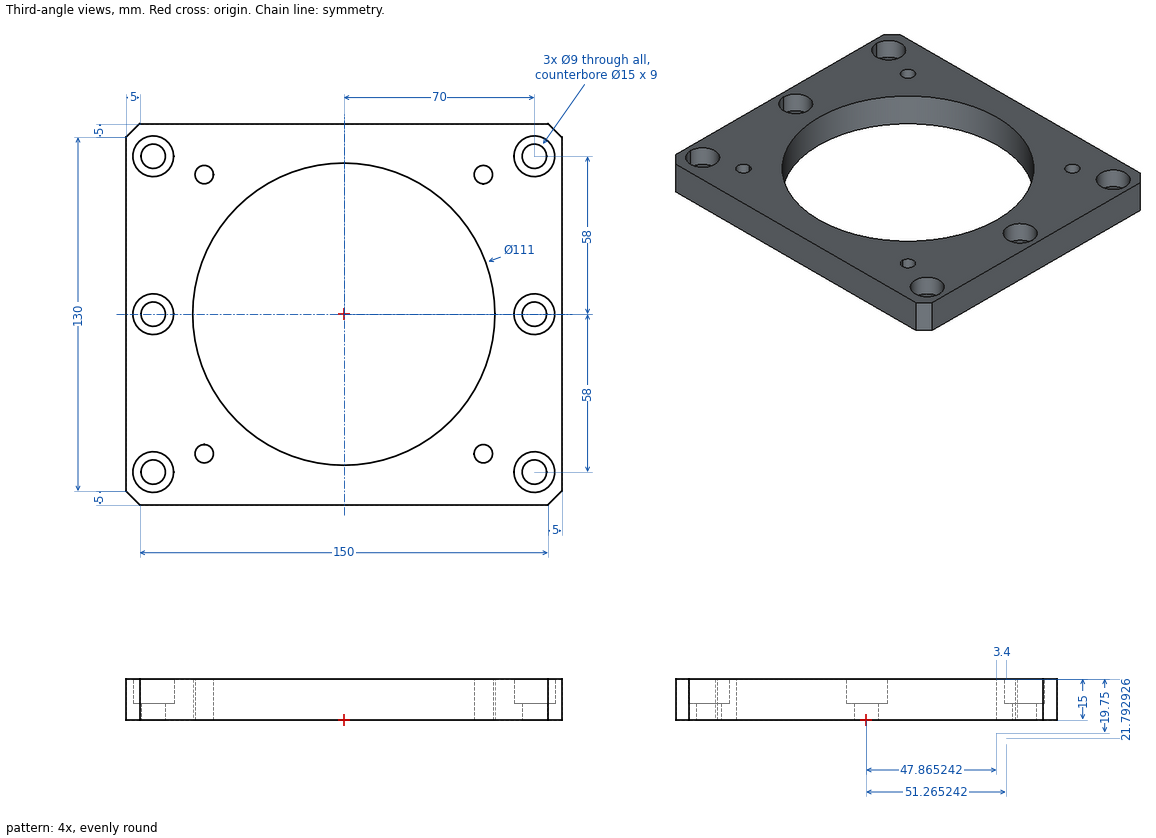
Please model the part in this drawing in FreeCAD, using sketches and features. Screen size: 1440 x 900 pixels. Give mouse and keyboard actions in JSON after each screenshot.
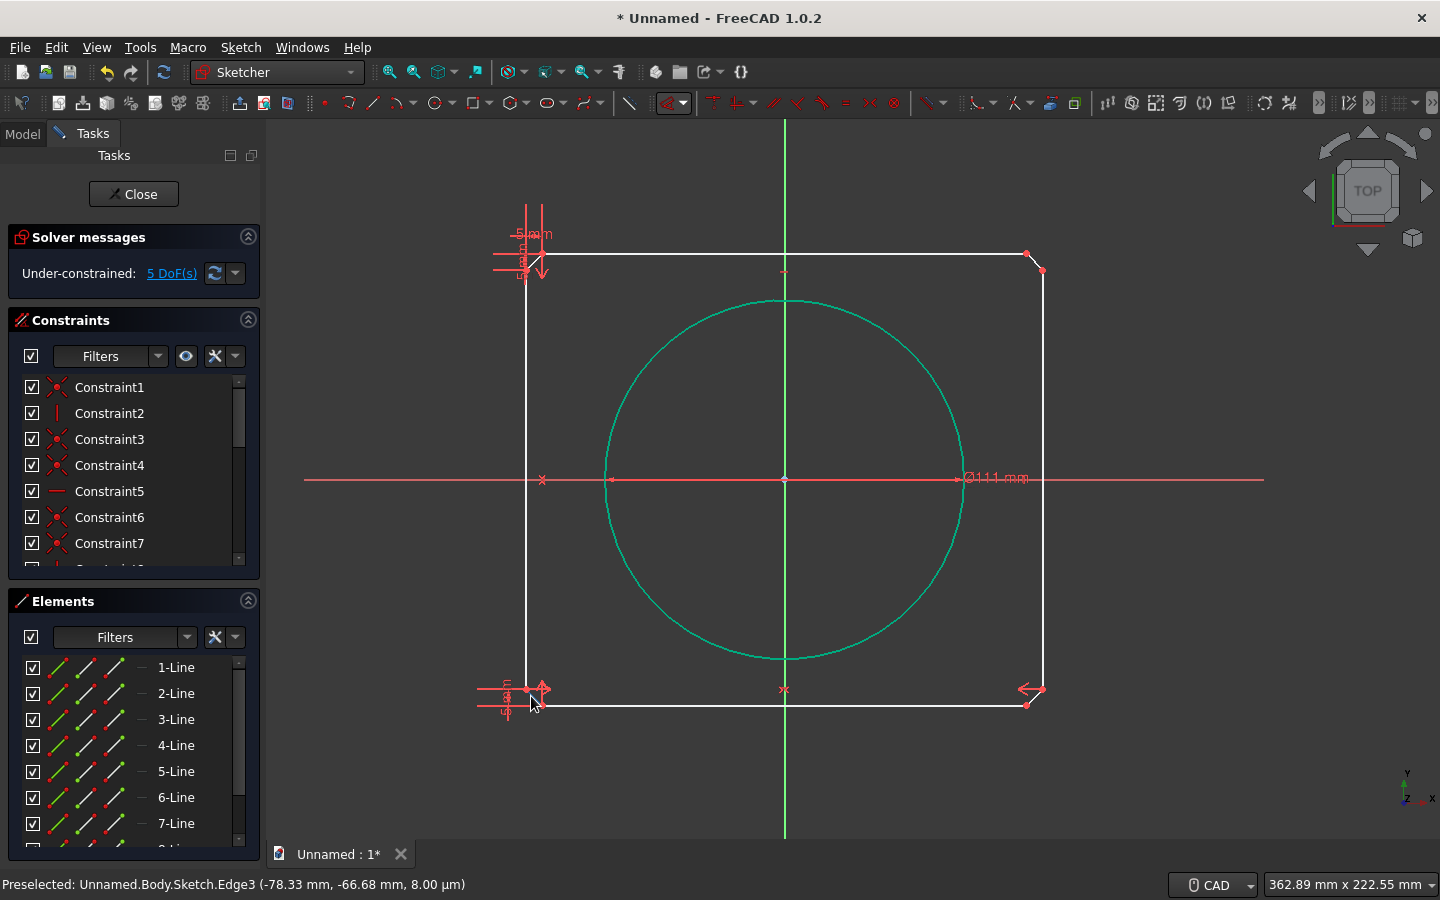
{"action": "scroll", "coordinate": [1032, 701], "scroll_direction": "up", "scroll_amount": 5}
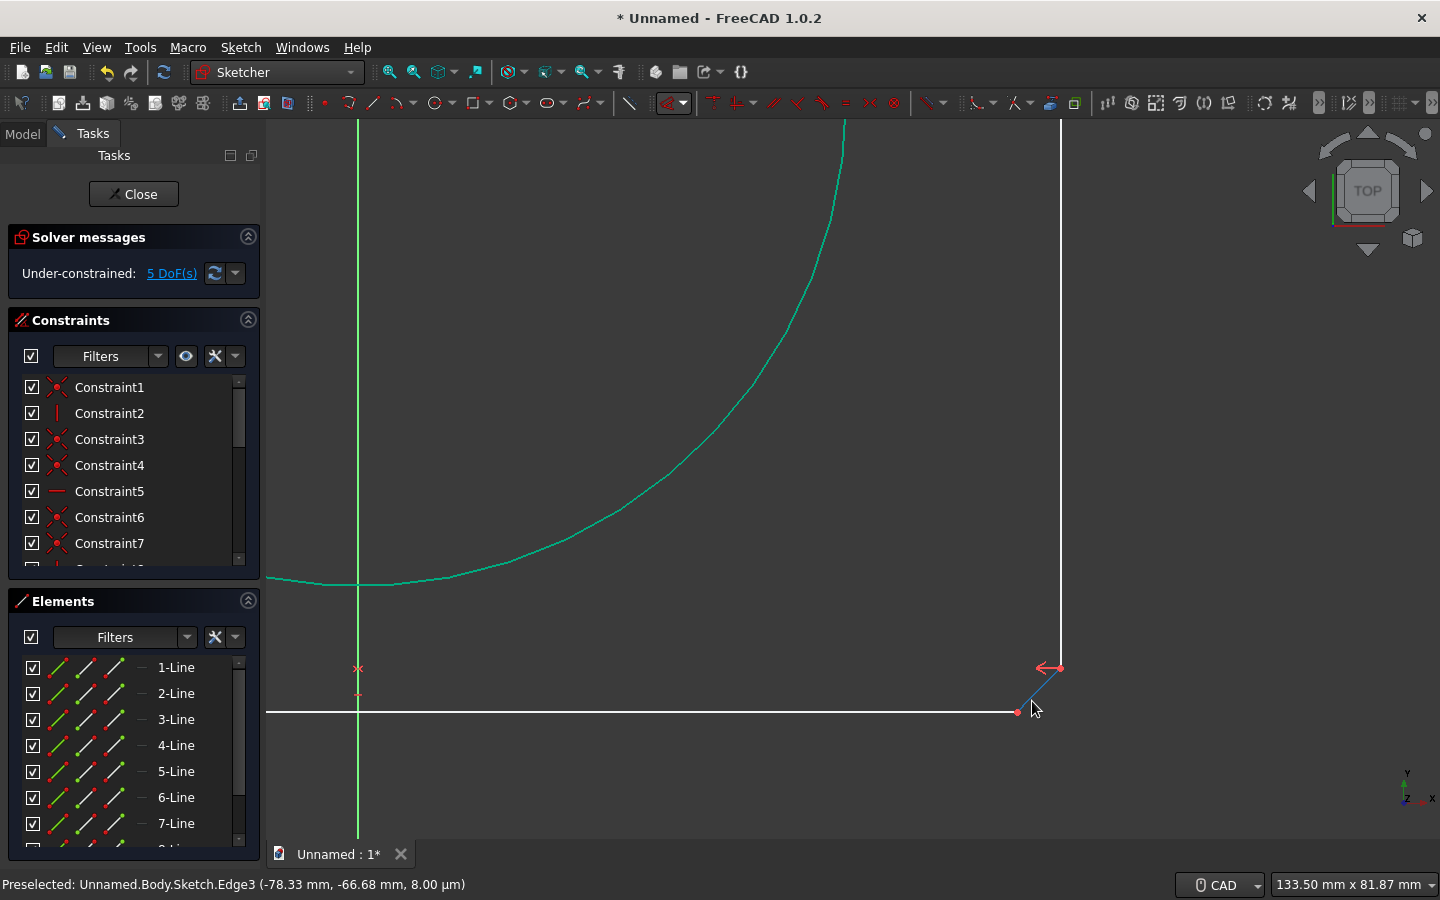
{"action": "left_click", "coordinate": [1030, 699]}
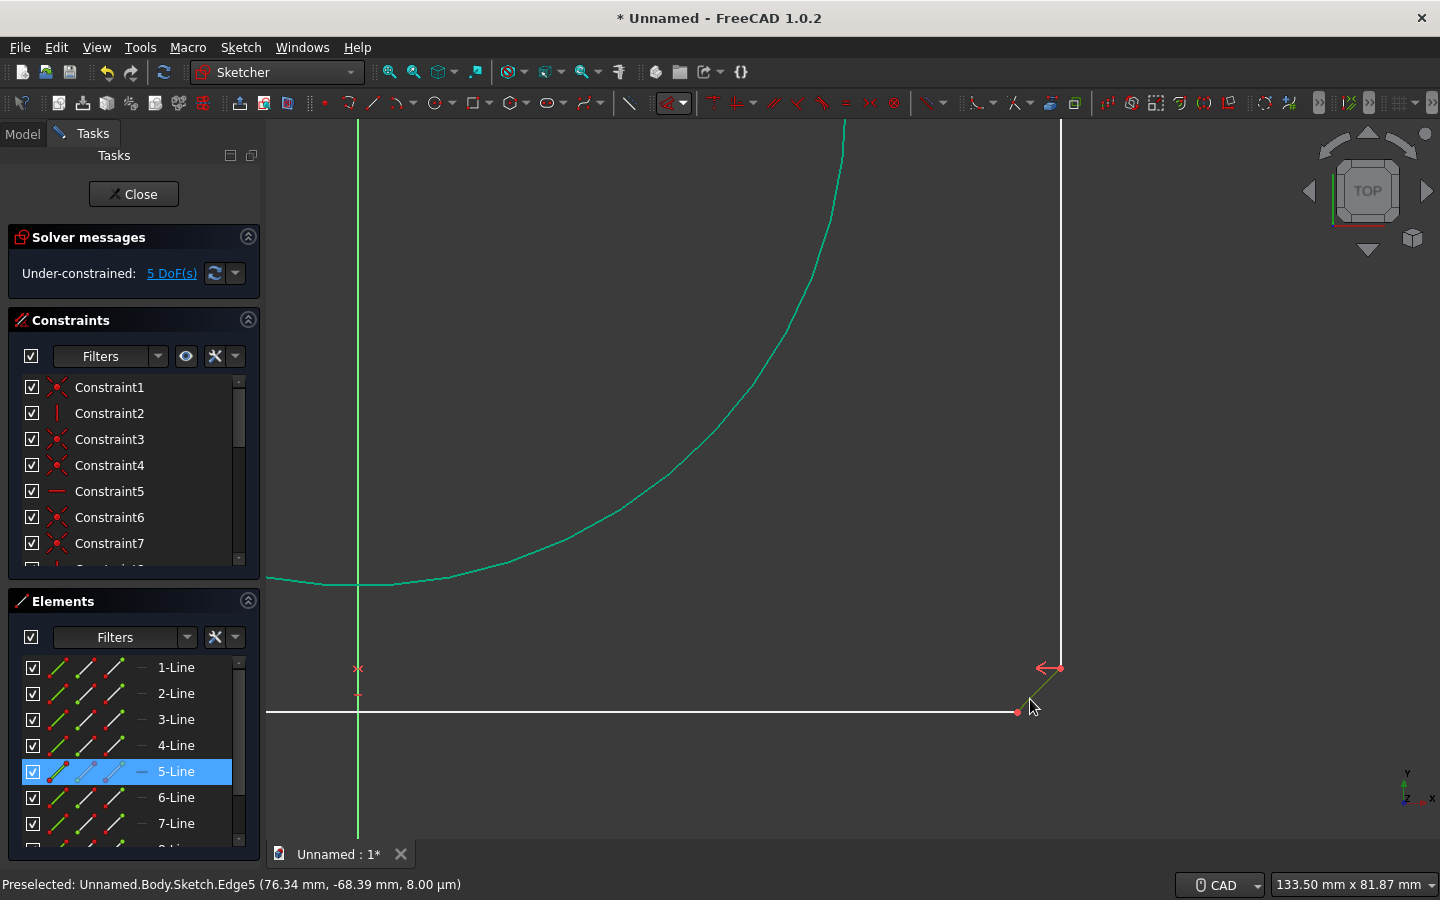
{"action": "left_click", "coordinate": [686, 104]}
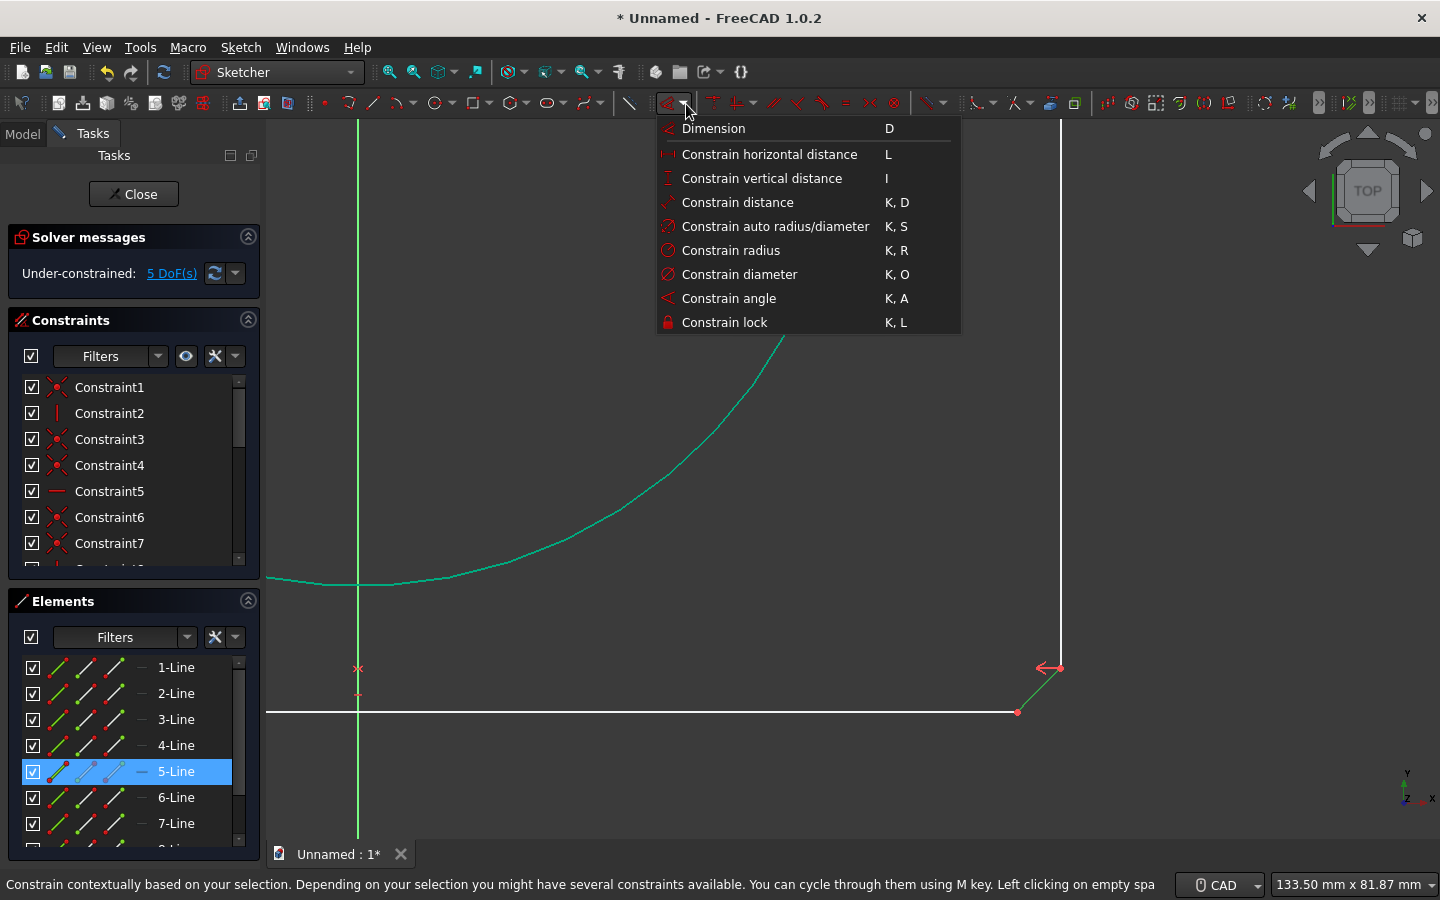
{"action": "left_click", "coordinate": [809, 154]}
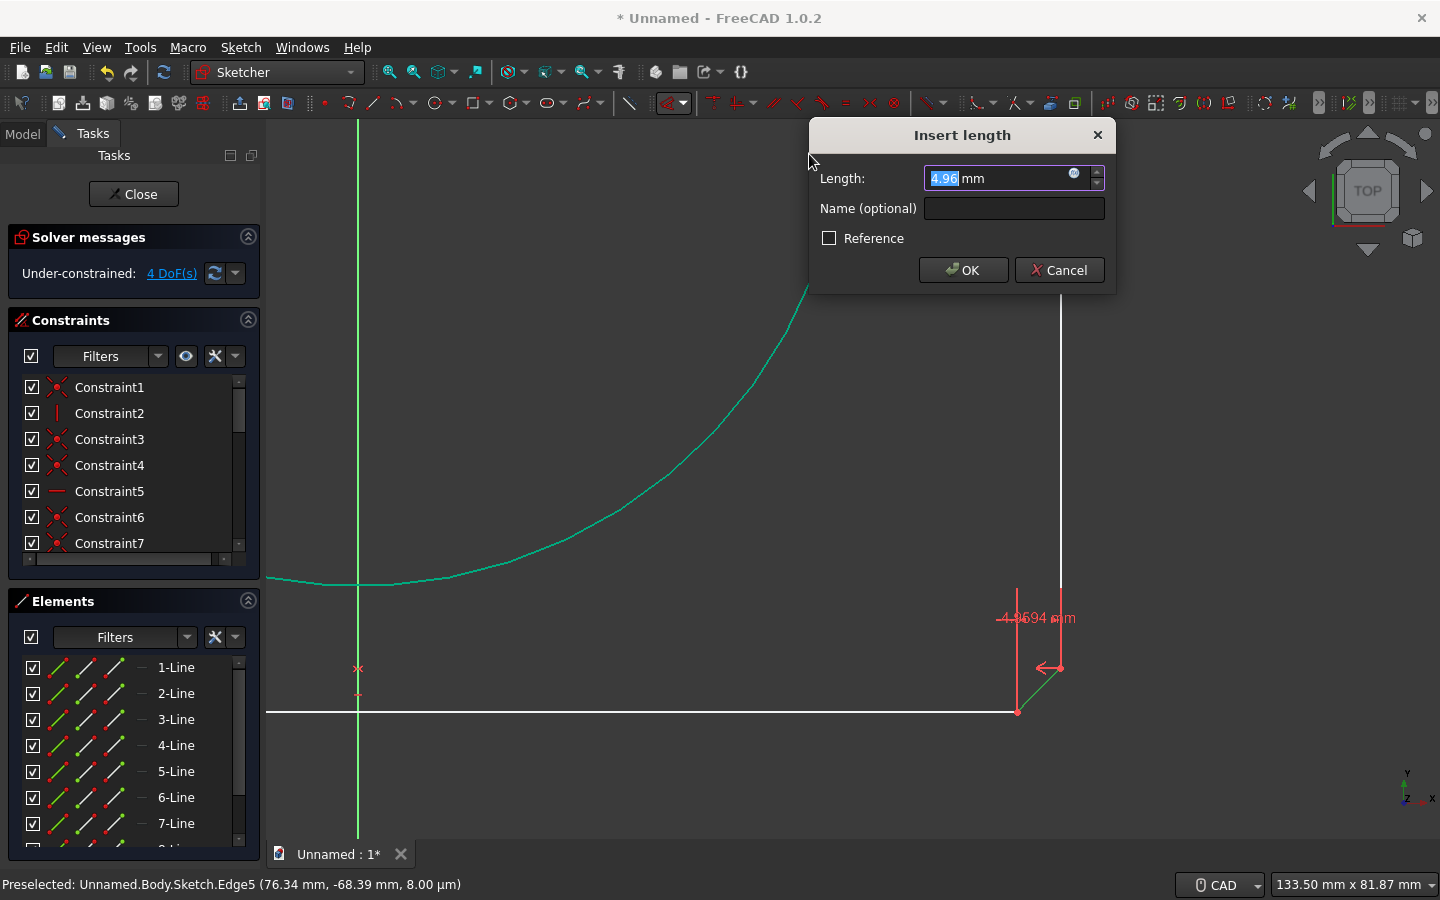
{"action": "type", "text": "5"}
{"action": "key", "text": "Return"}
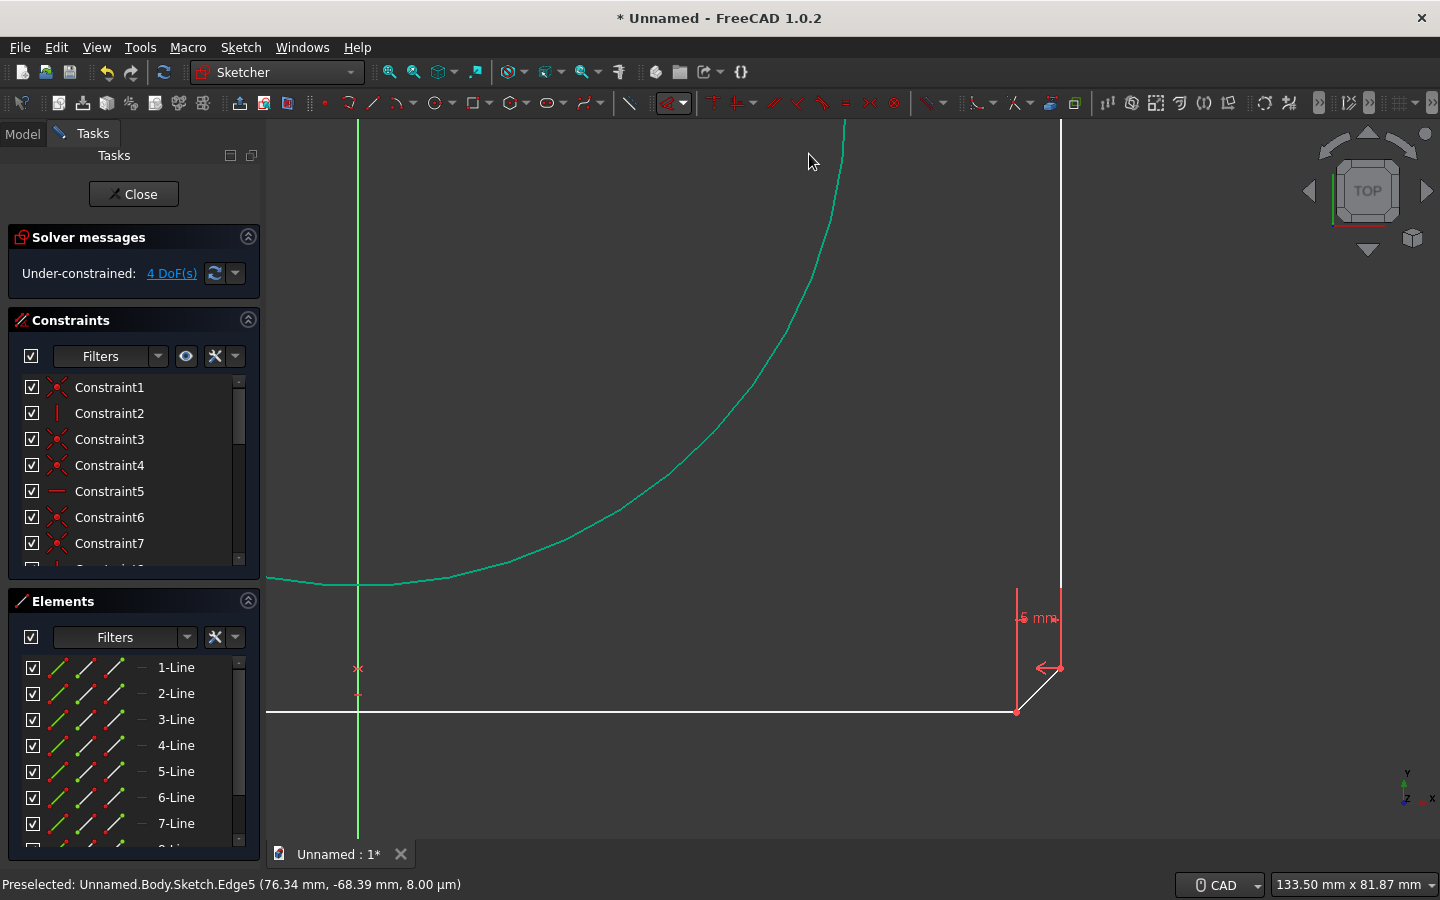
{"action": "scroll", "coordinate": [1033, 701], "scroll_direction": "down", "scroll_amount": 5}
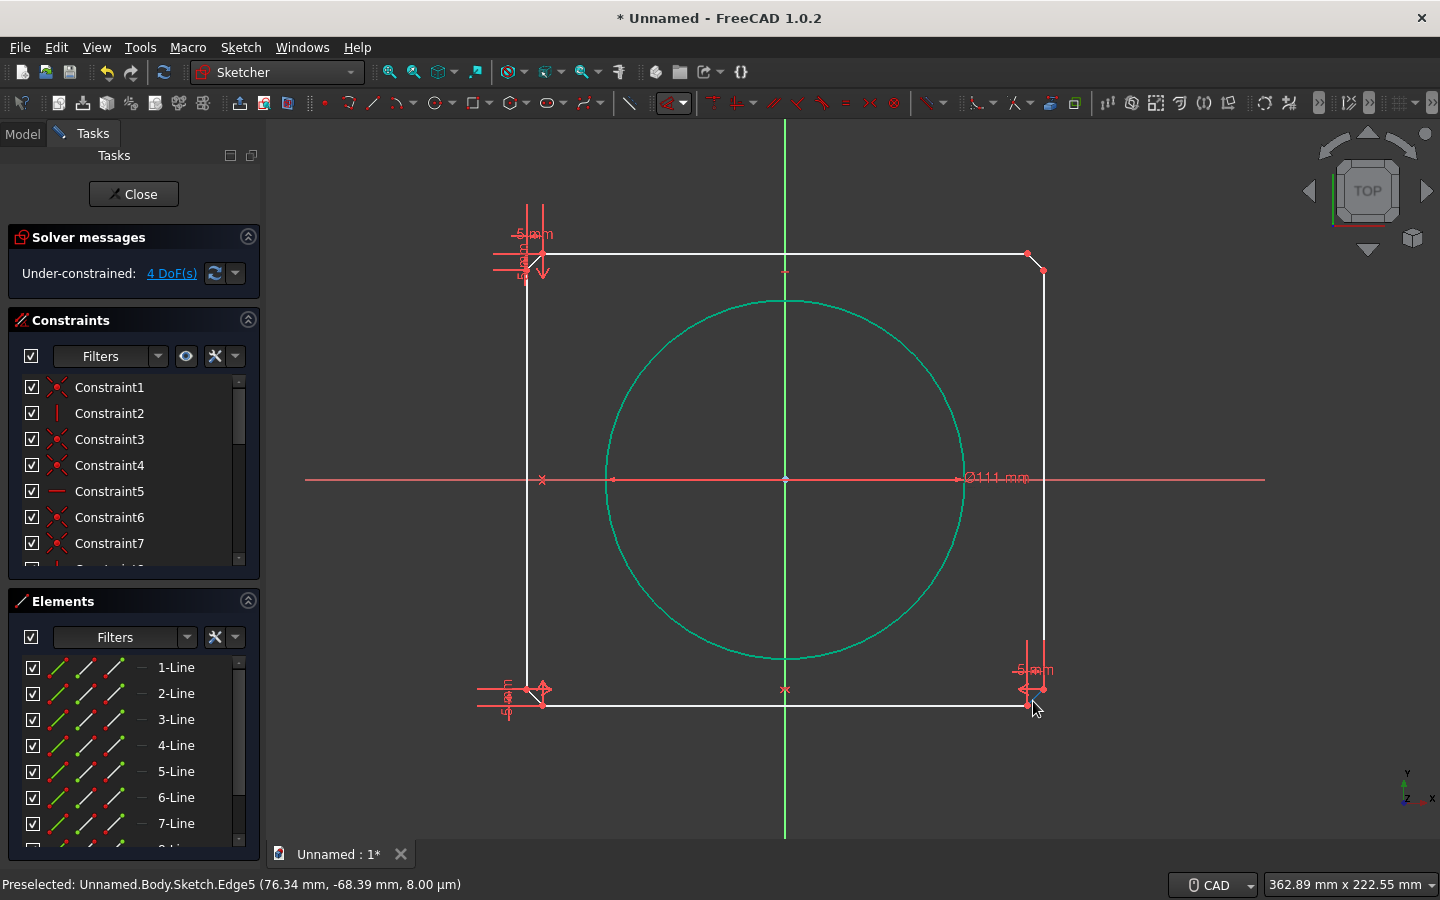
{"action": "scroll", "coordinate": [1039, 265], "scroll_direction": "up", "scroll_amount": 5}